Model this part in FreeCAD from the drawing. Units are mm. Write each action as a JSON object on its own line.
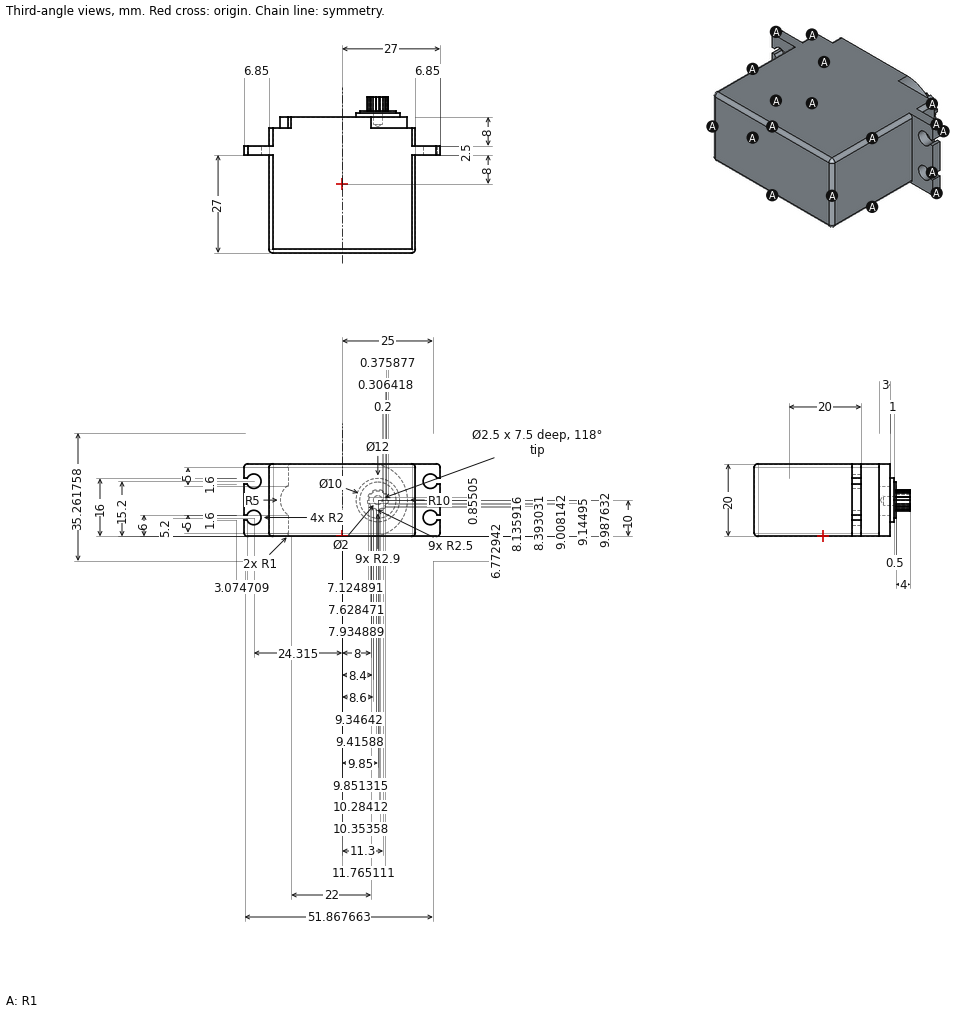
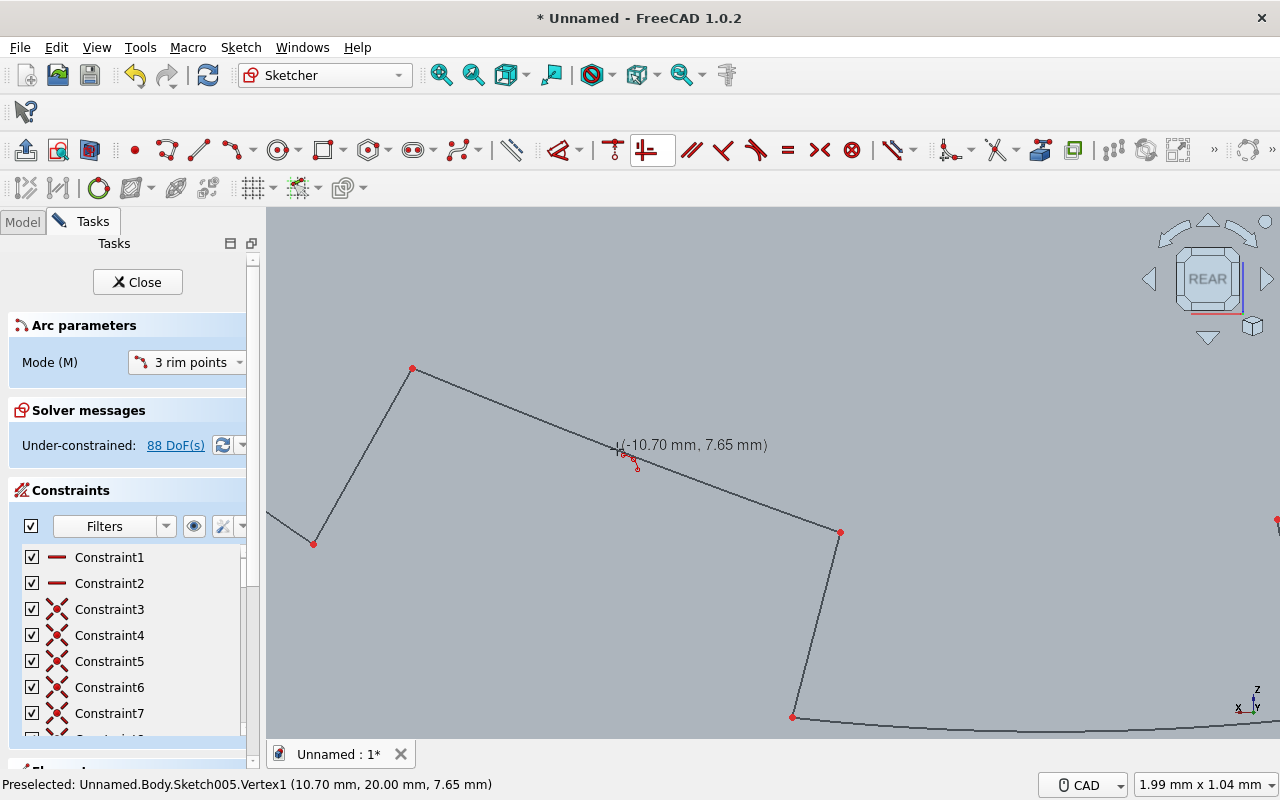
{"action": "left_click", "coordinate": [278, 150]}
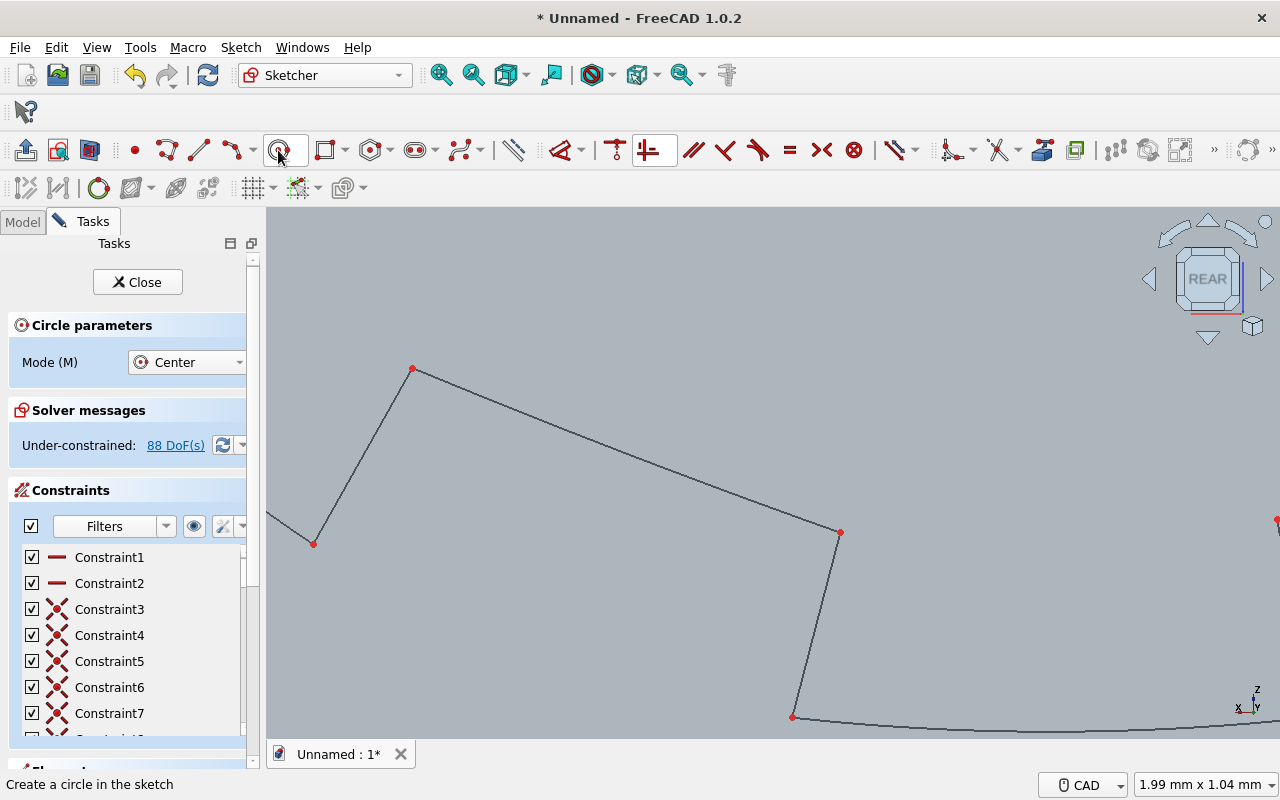
{"action": "scroll", "coordinate": [593, 442], "scroll_direction": "down", "scroll_amount": 15}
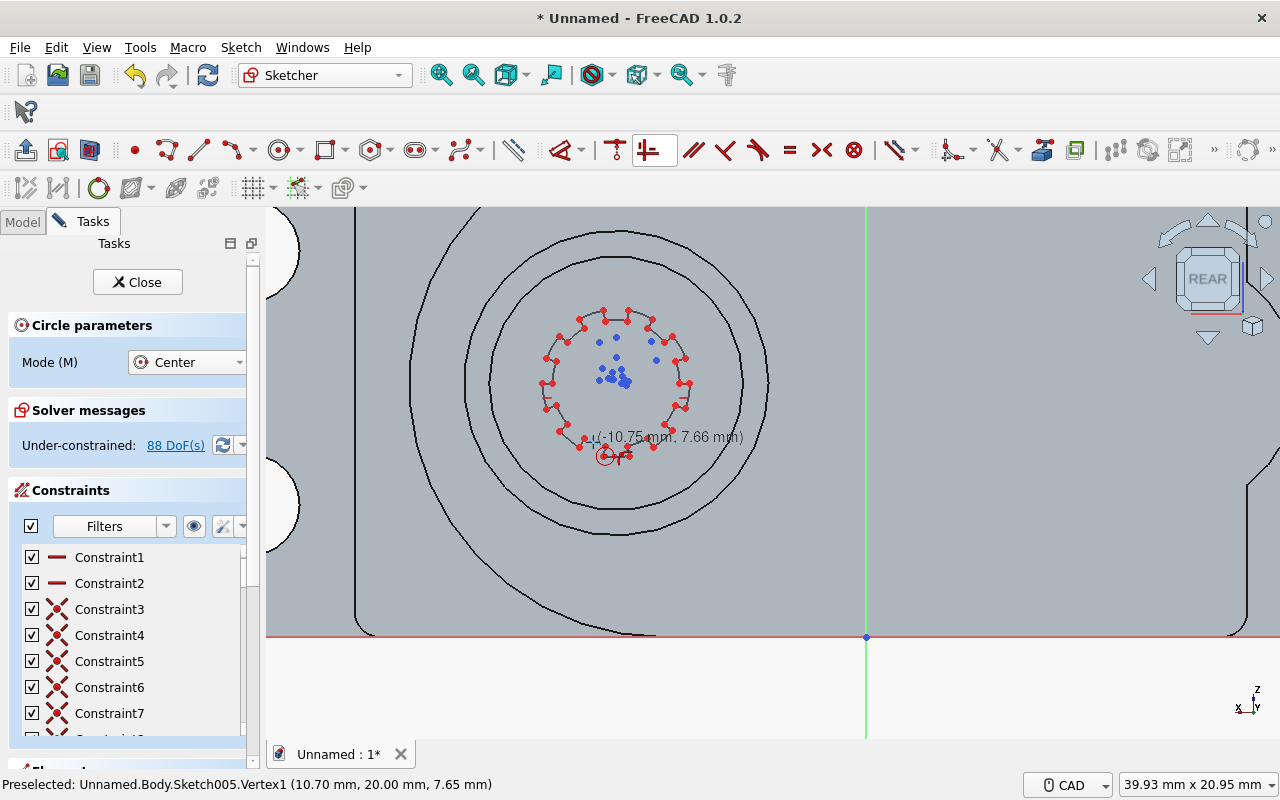
{"action": "left_click", "coordinate": [616, 383]}
{"action": "mouse_move", "coordinate": [634, 365]}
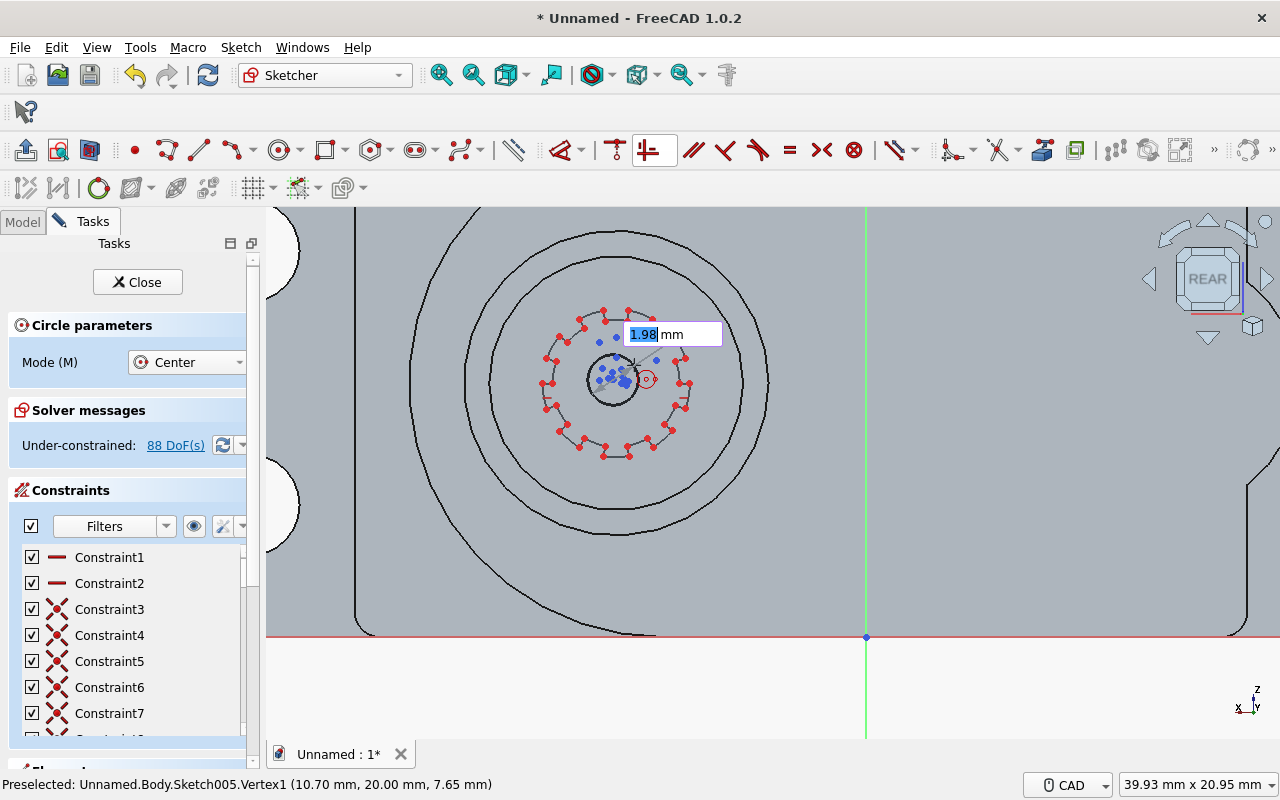
{"action": "type", "text": "2"}
{"action": "key", "text": "Return"}
{"action": "key", "text": "Escape"}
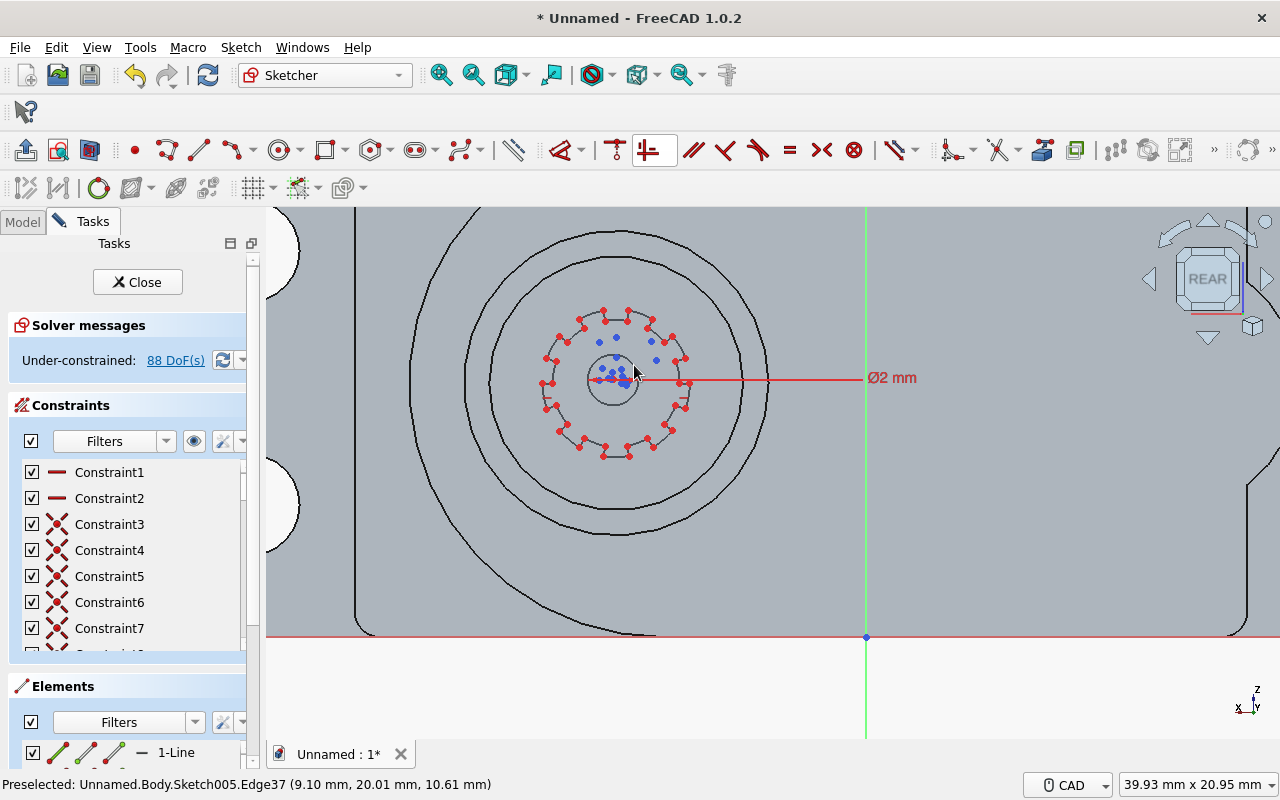
{"action": "left_click", "coordinate": [631, 362]}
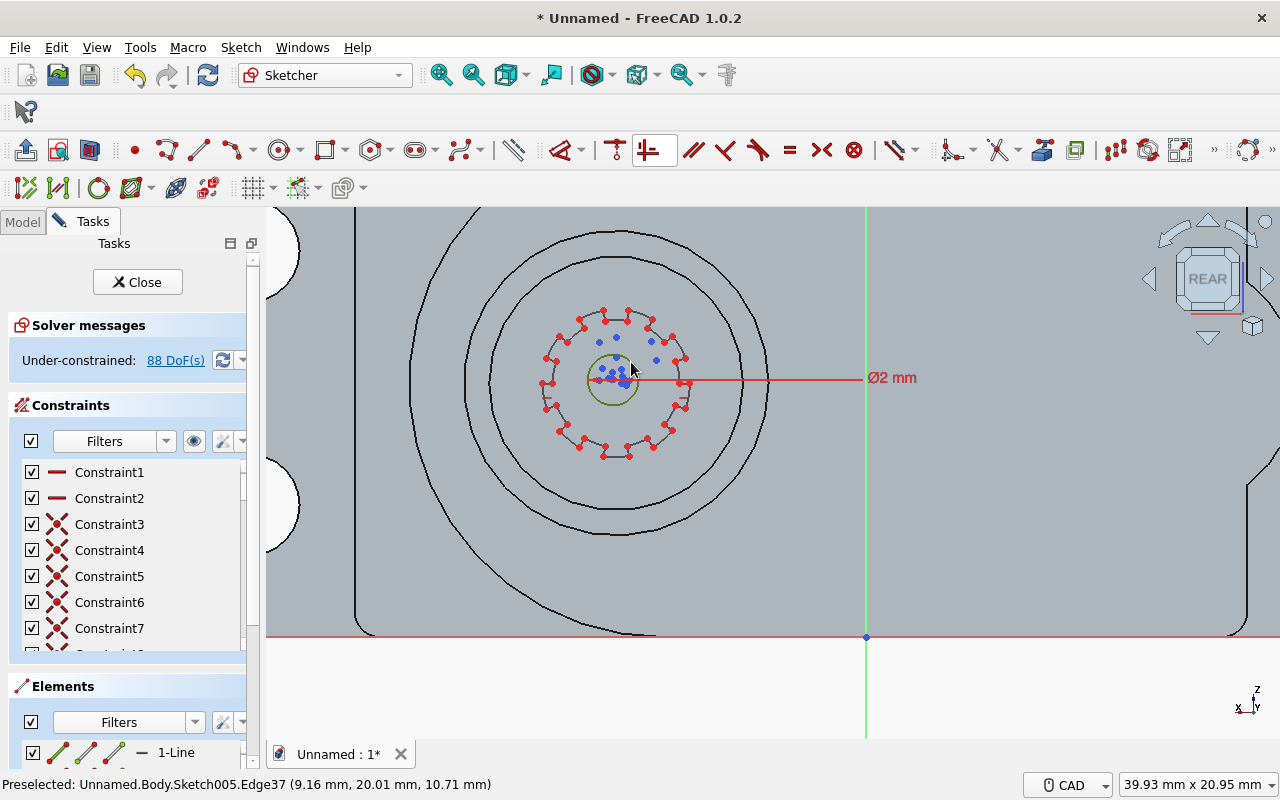
{"action": "left_click", "coordinate": [616, 457]}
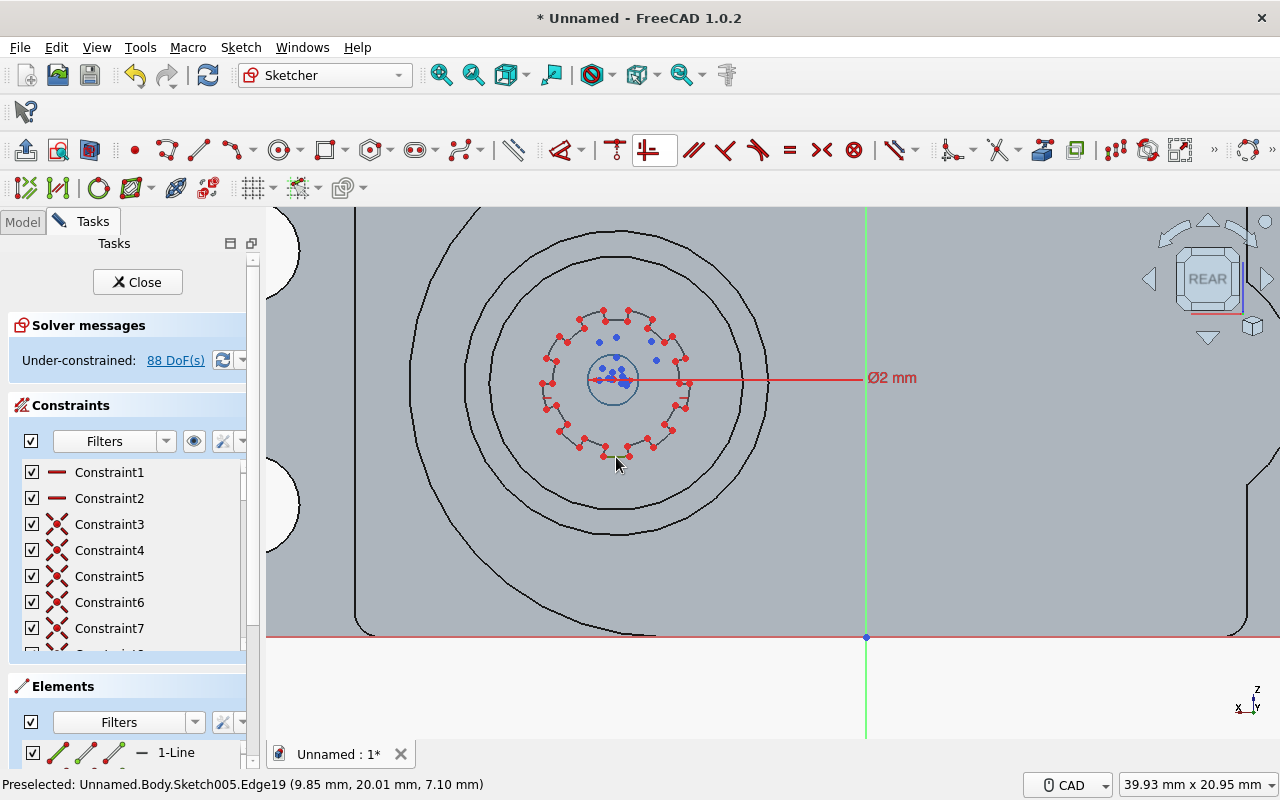
{"action": "key", "text": "c"}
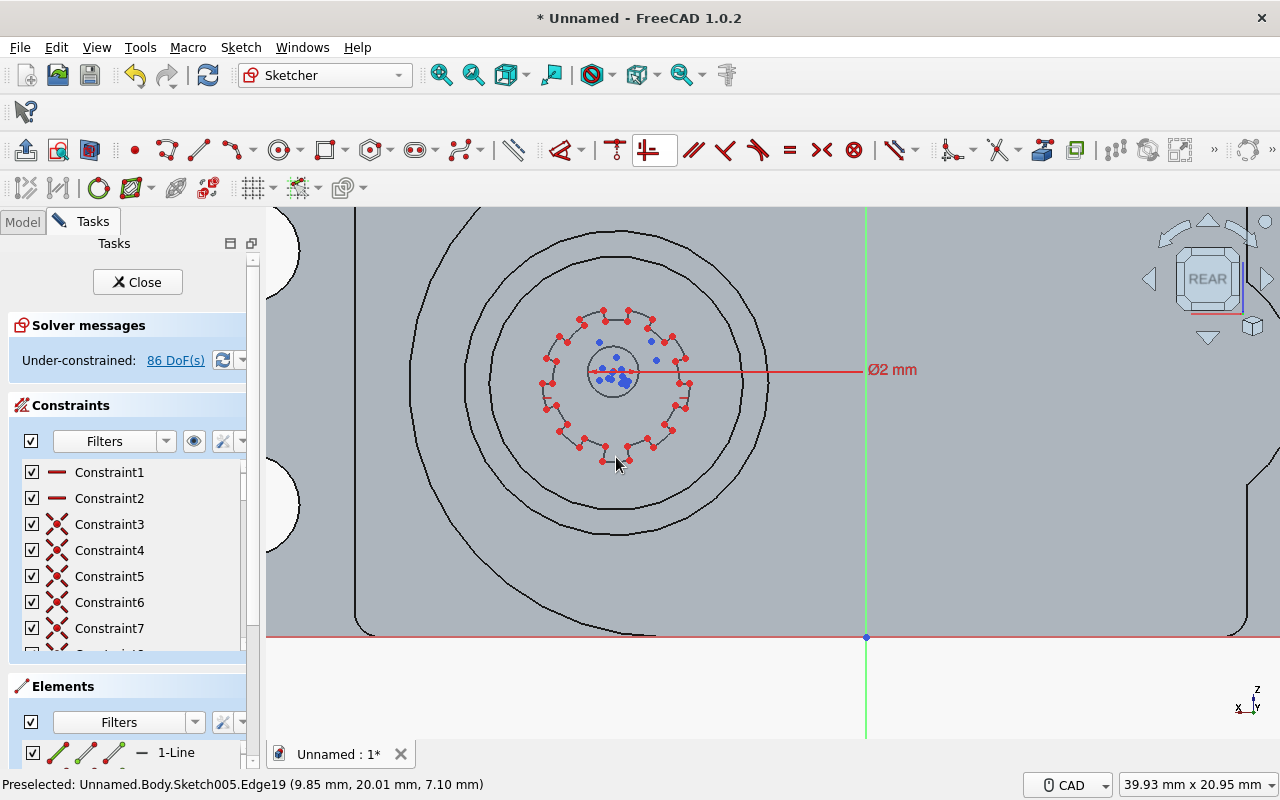
{"action": "left_click", "coordinate": [631, 354]}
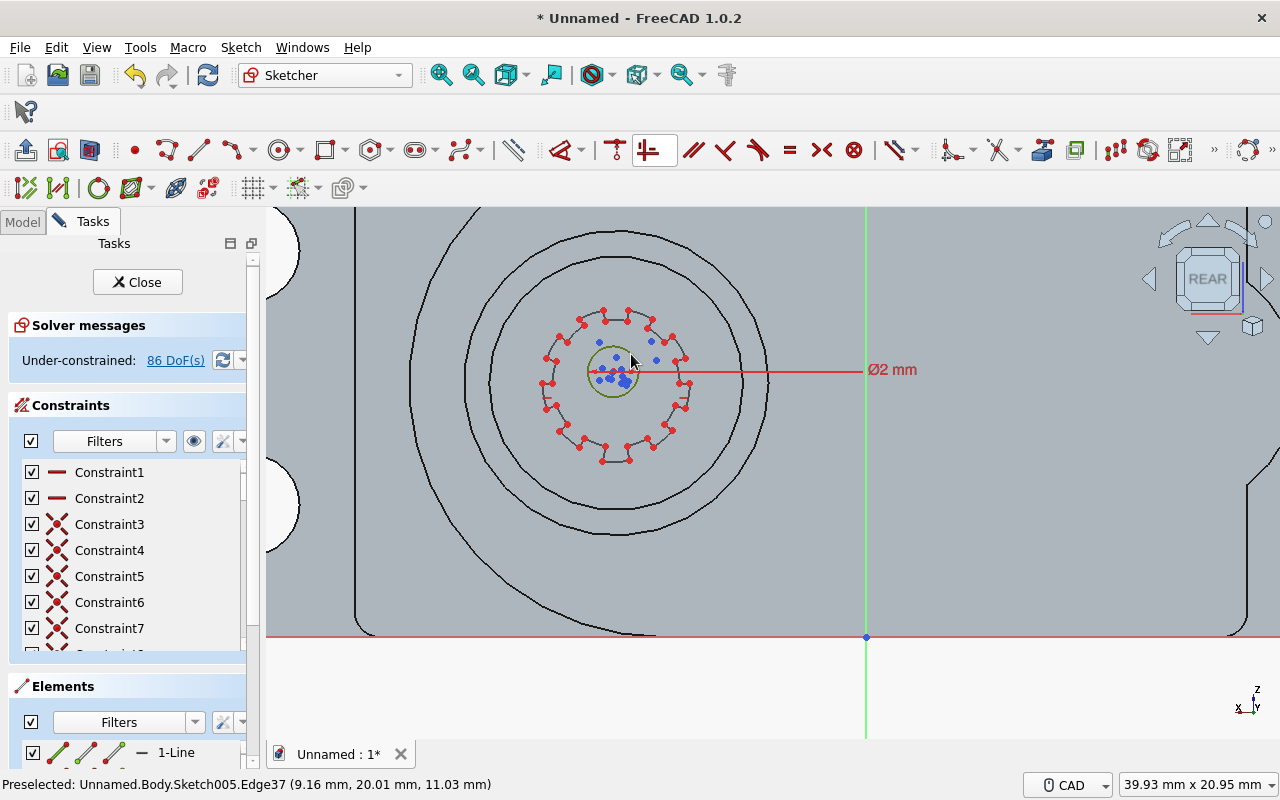
{"action": "scroll", "coordinate": [638, 443], "scroll_direction": "up", "scroll_amount": 2}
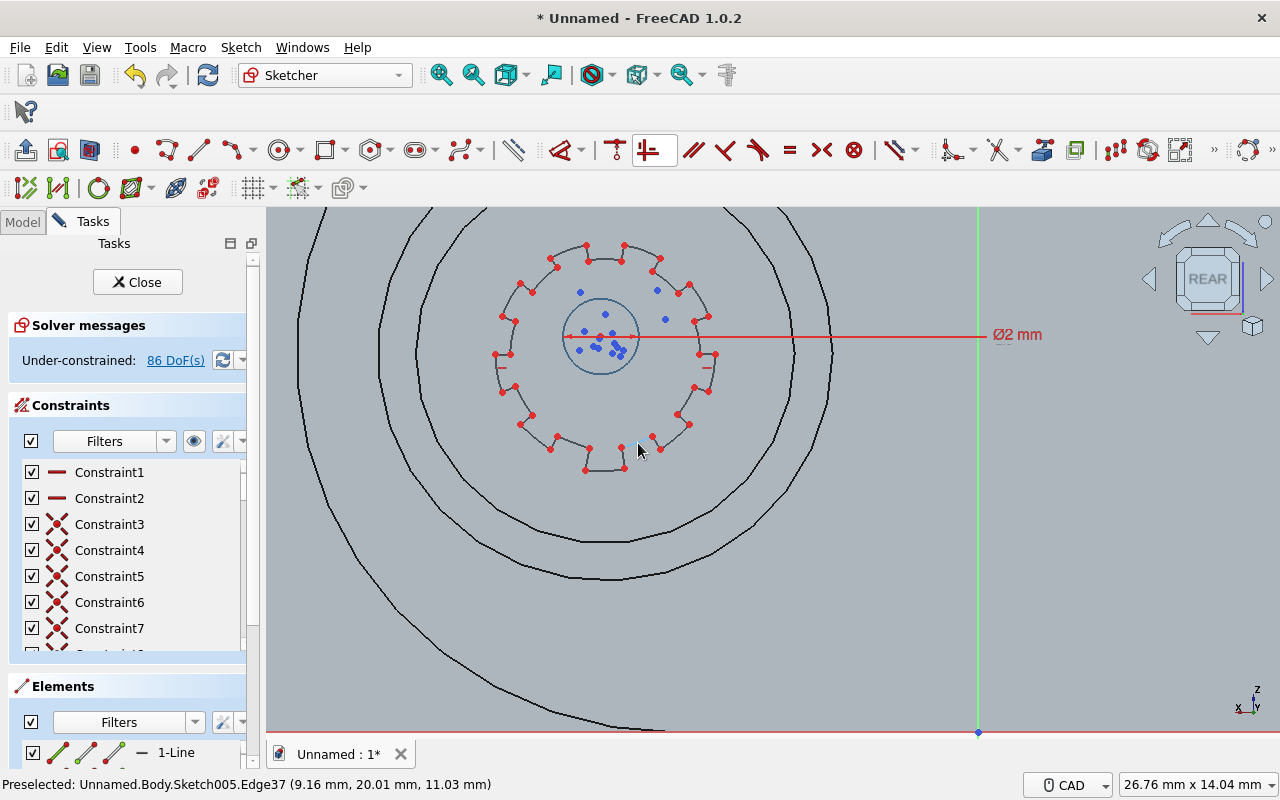
{"action": "left_click", "coordinate": [637, 443]}